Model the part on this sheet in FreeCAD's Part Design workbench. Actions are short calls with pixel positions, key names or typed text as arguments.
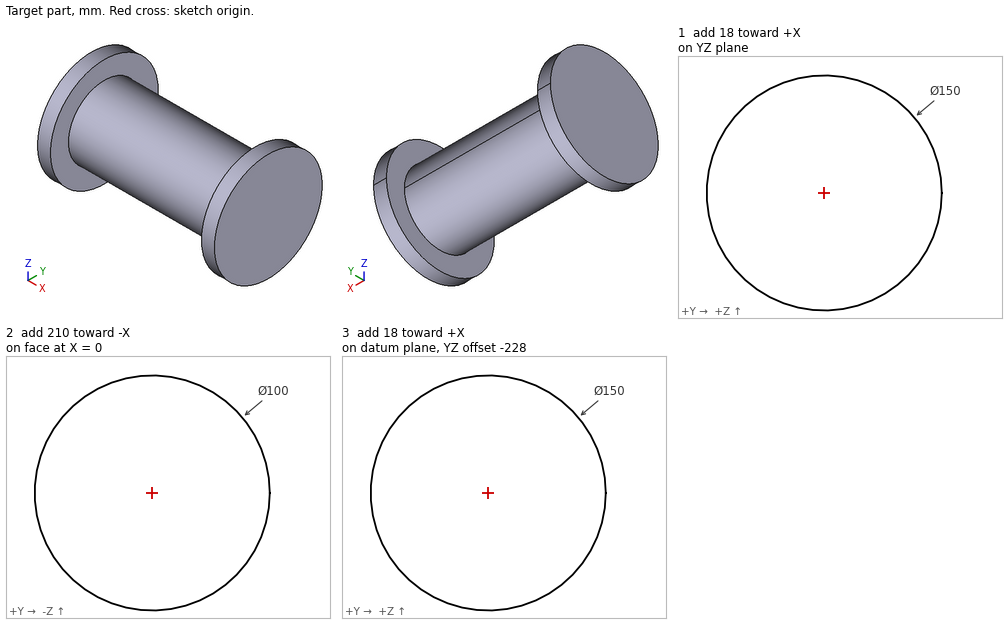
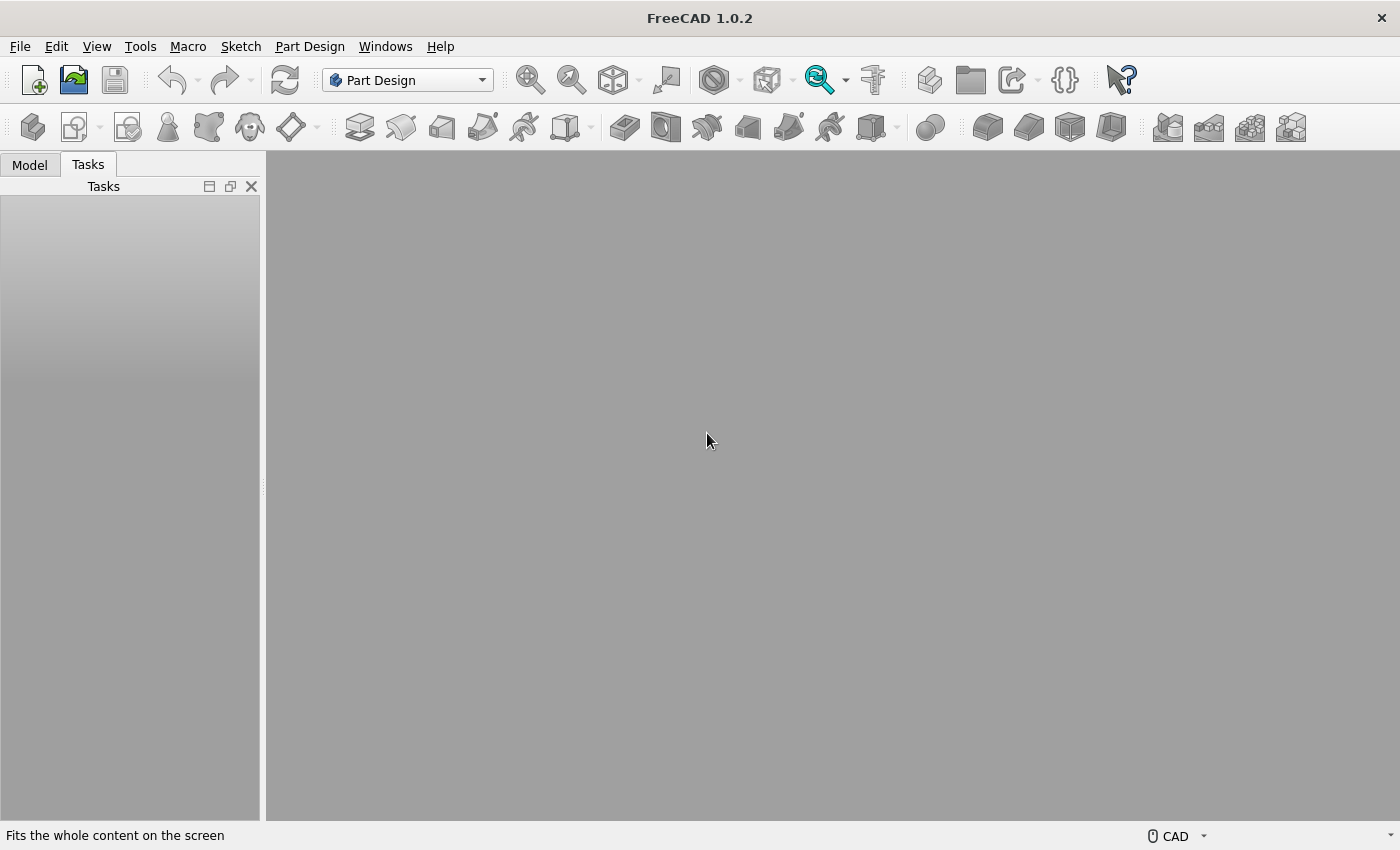
key(ctrl+n)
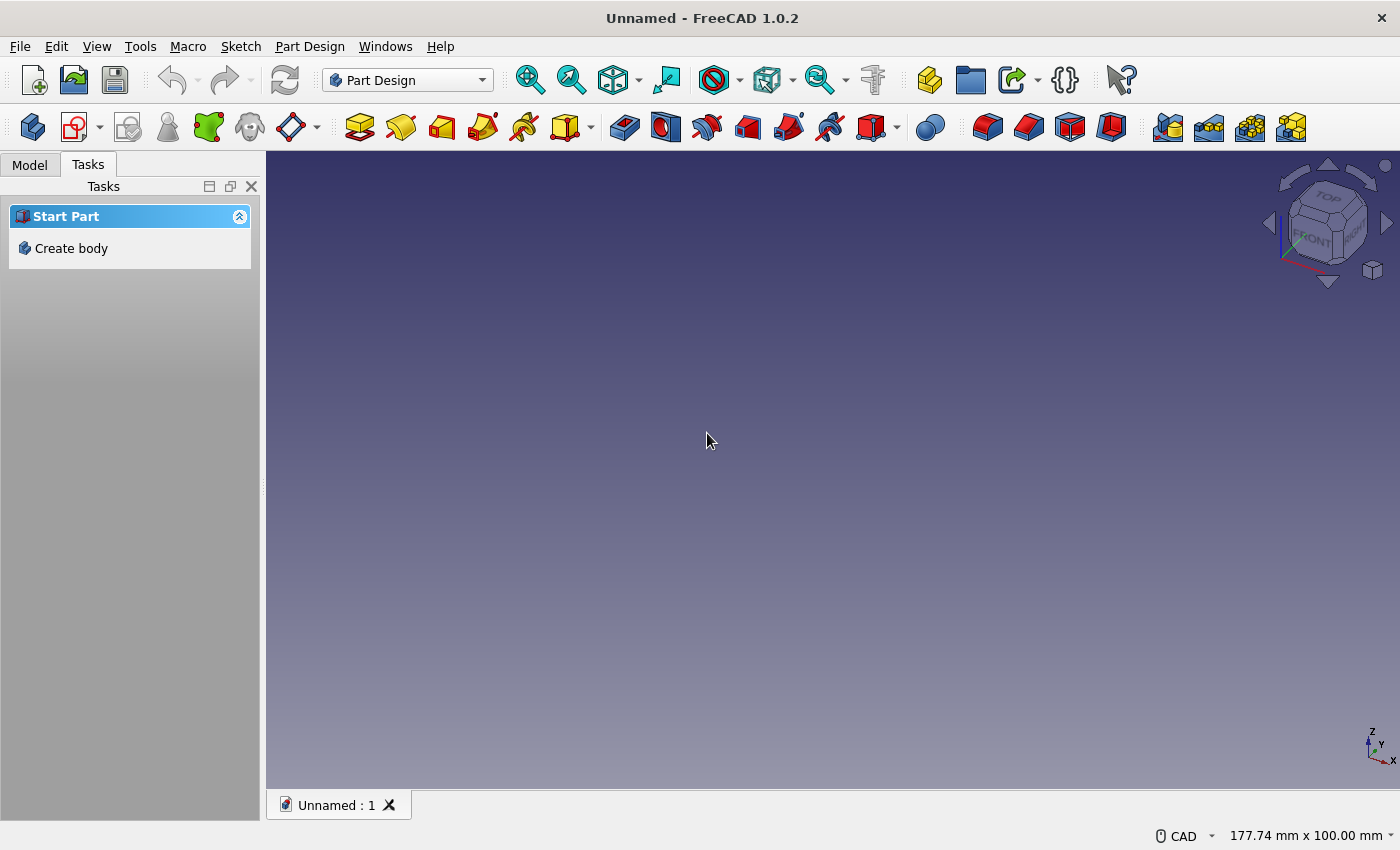
click(74, 128)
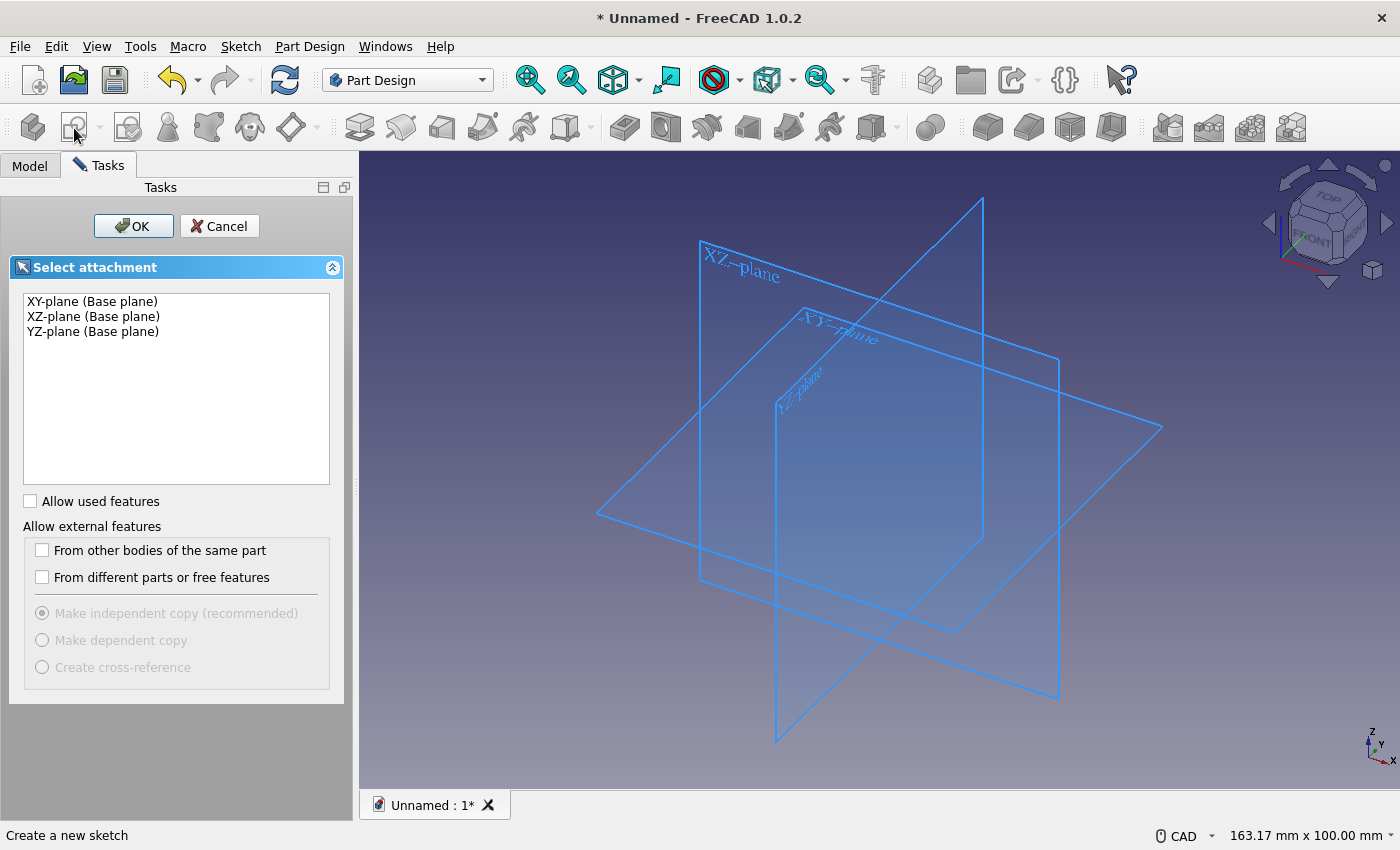
click(84, 332)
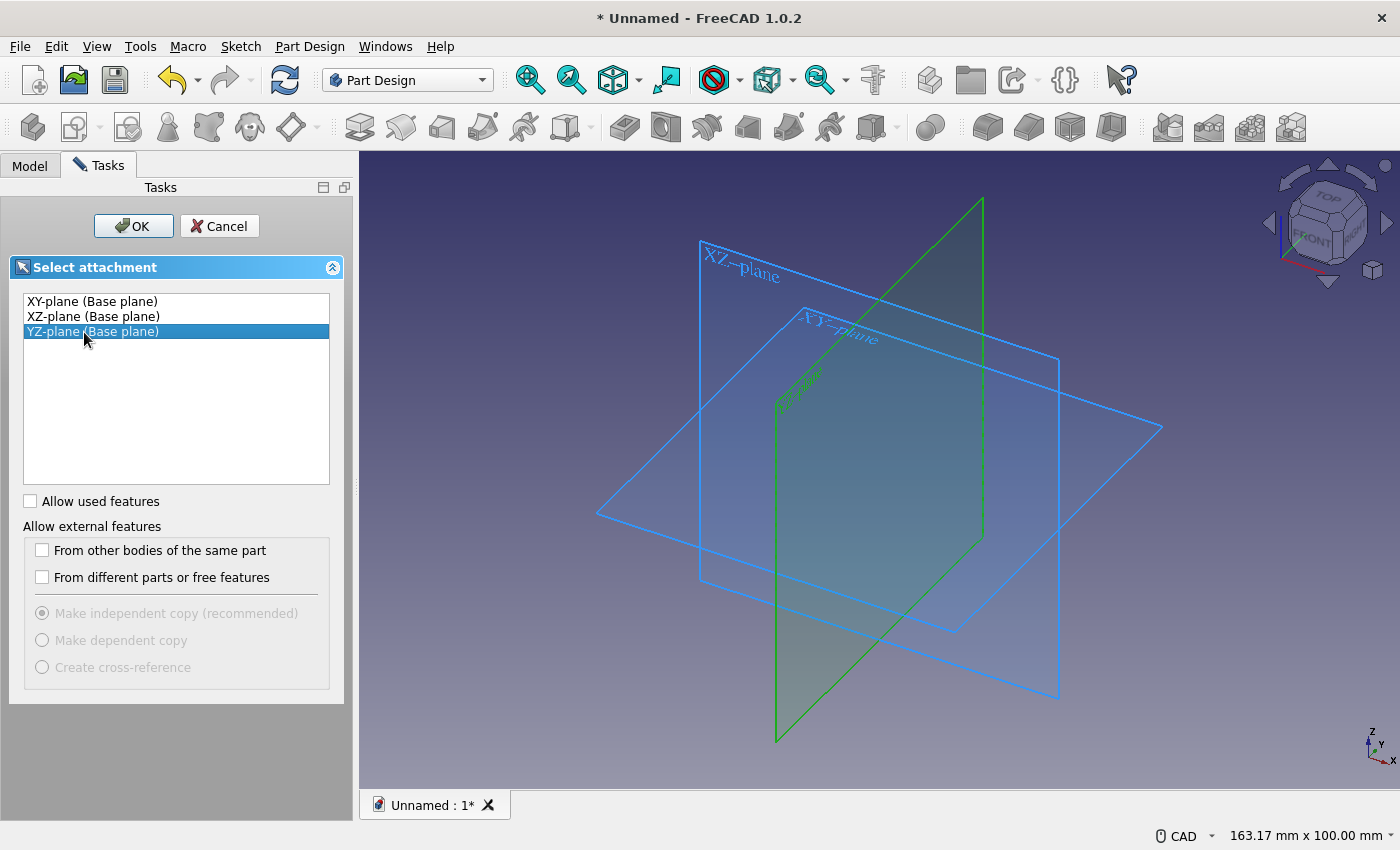
click(134, 226)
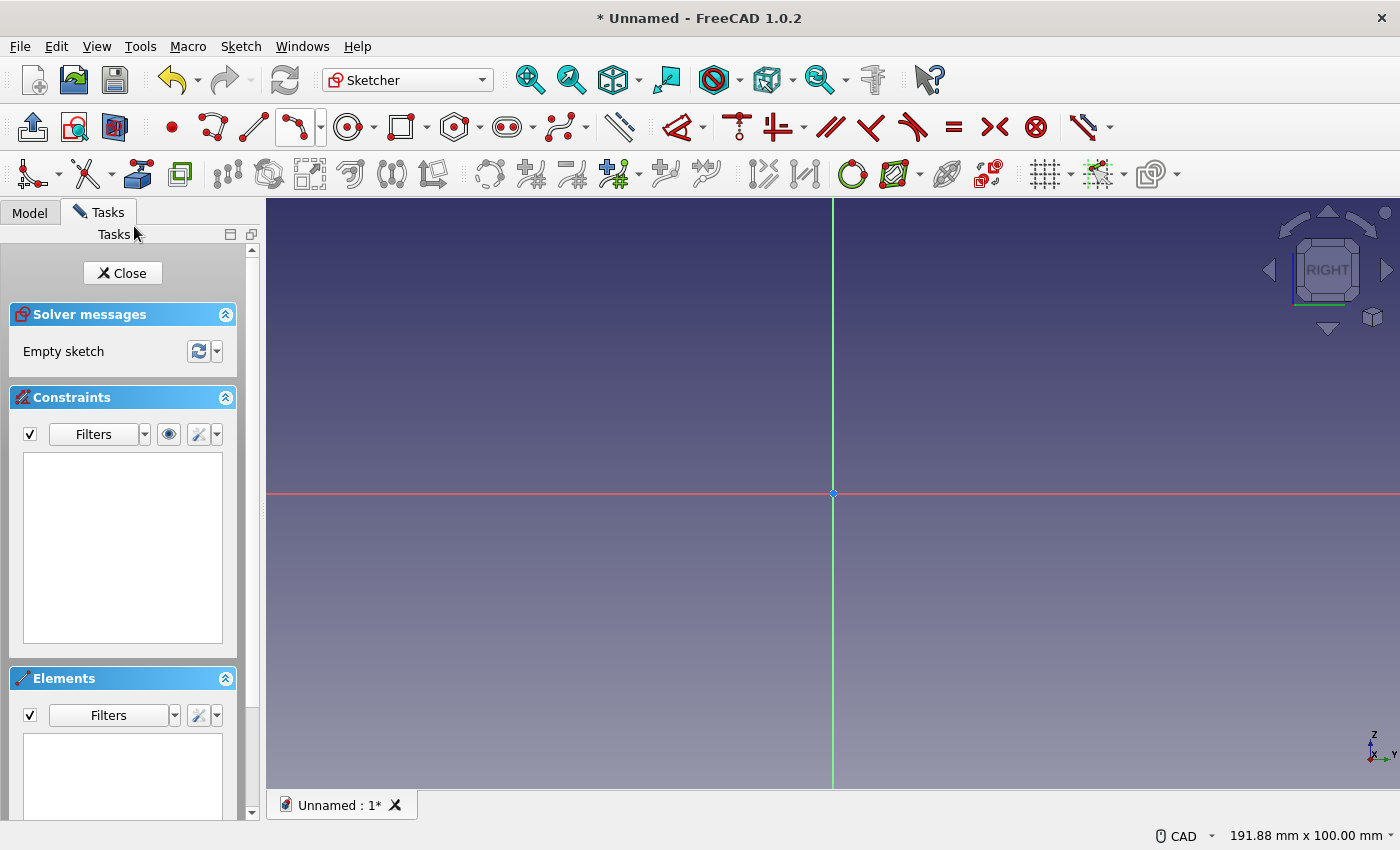
scroll(709, 494, down, 4)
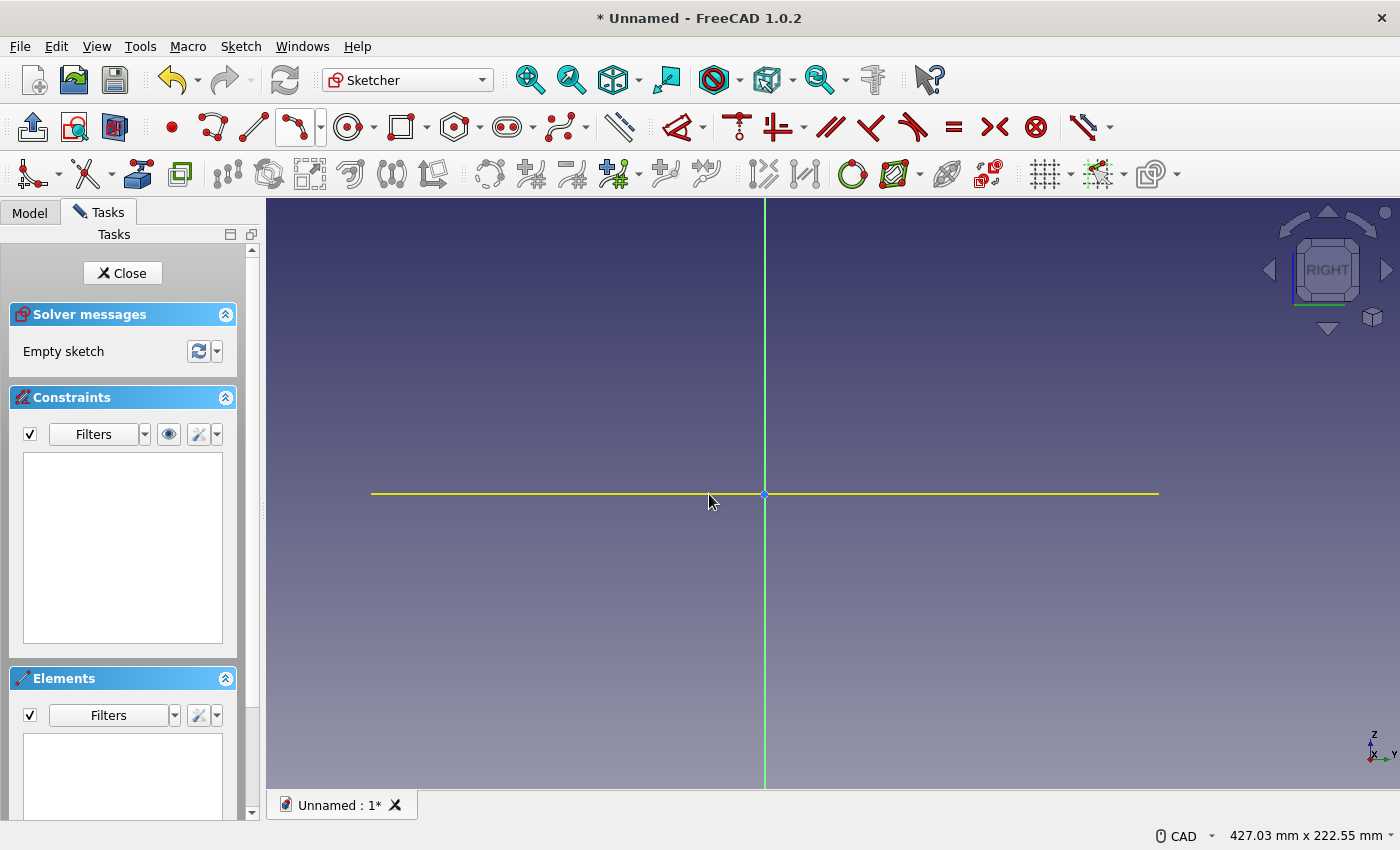
click(348, 128)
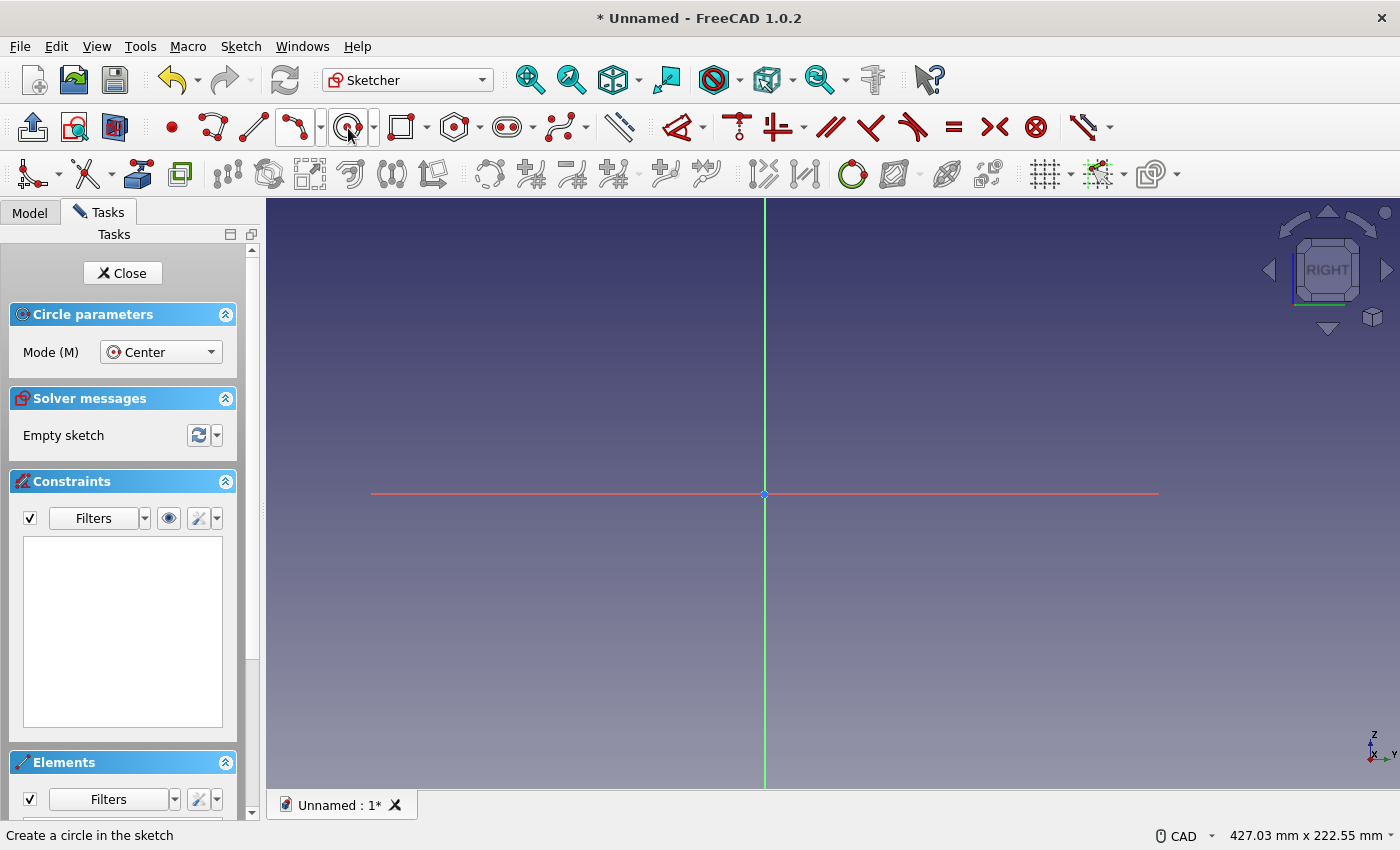
click(765, 494)
move(906, 353)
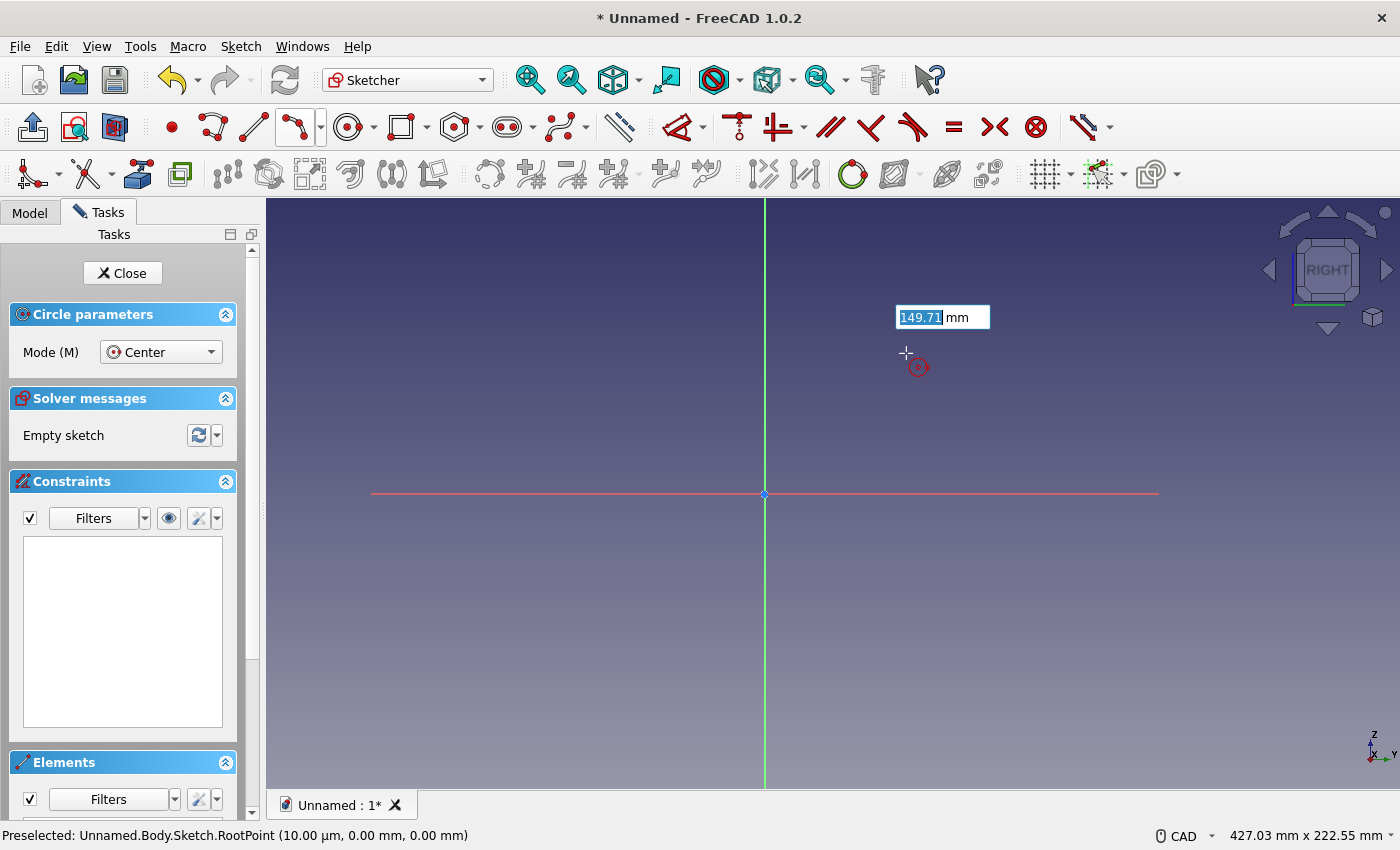
text(150)
key(Return)
key(Escape)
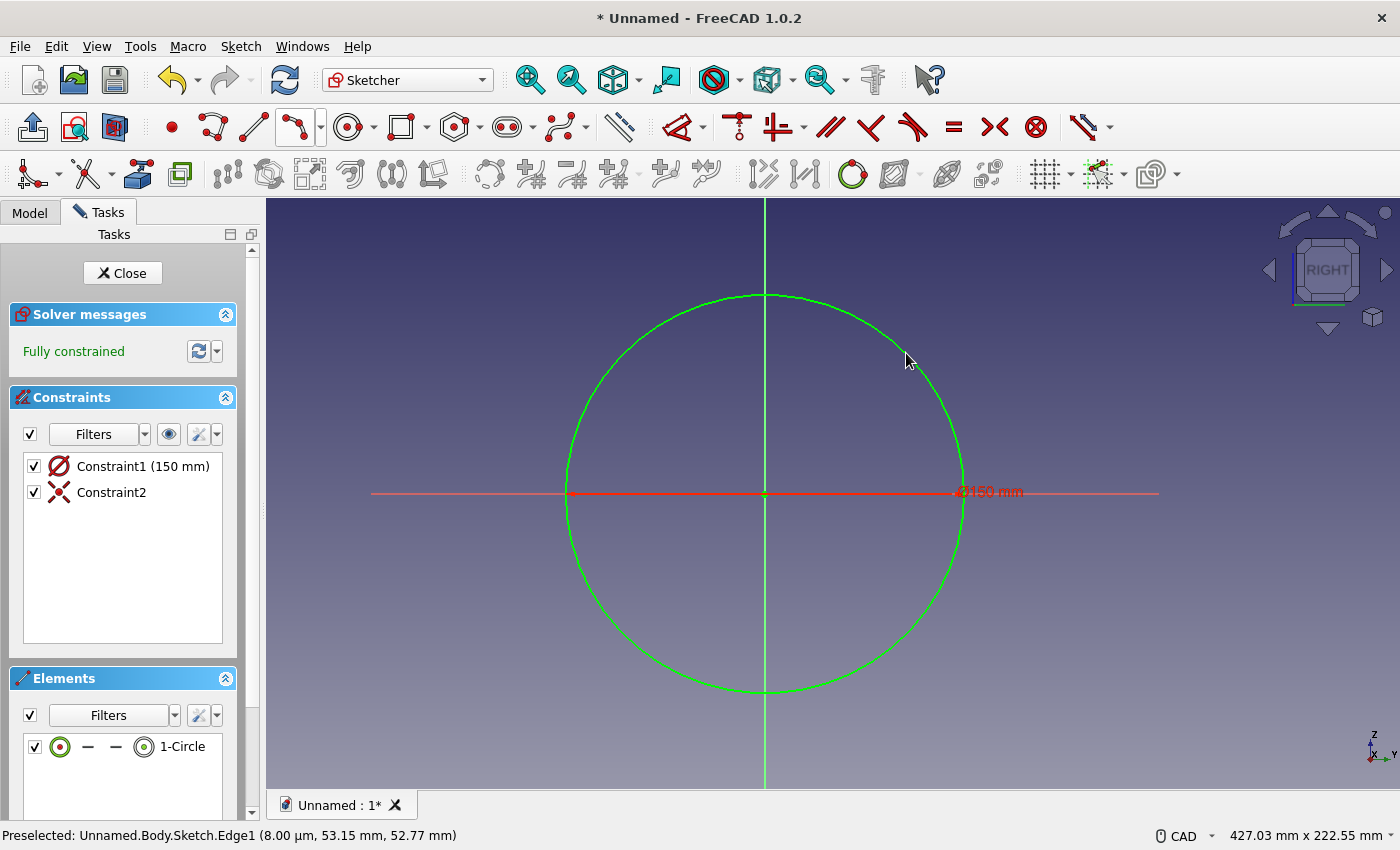
click(123, 273)